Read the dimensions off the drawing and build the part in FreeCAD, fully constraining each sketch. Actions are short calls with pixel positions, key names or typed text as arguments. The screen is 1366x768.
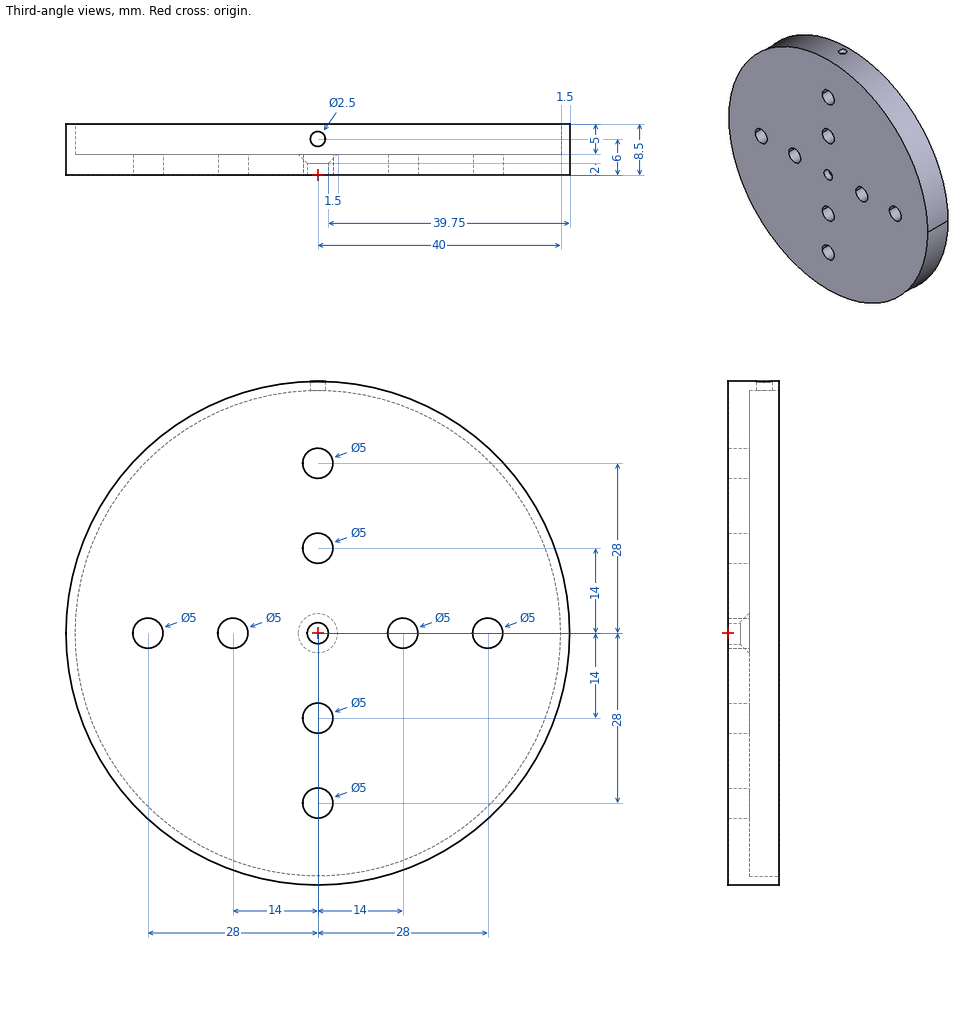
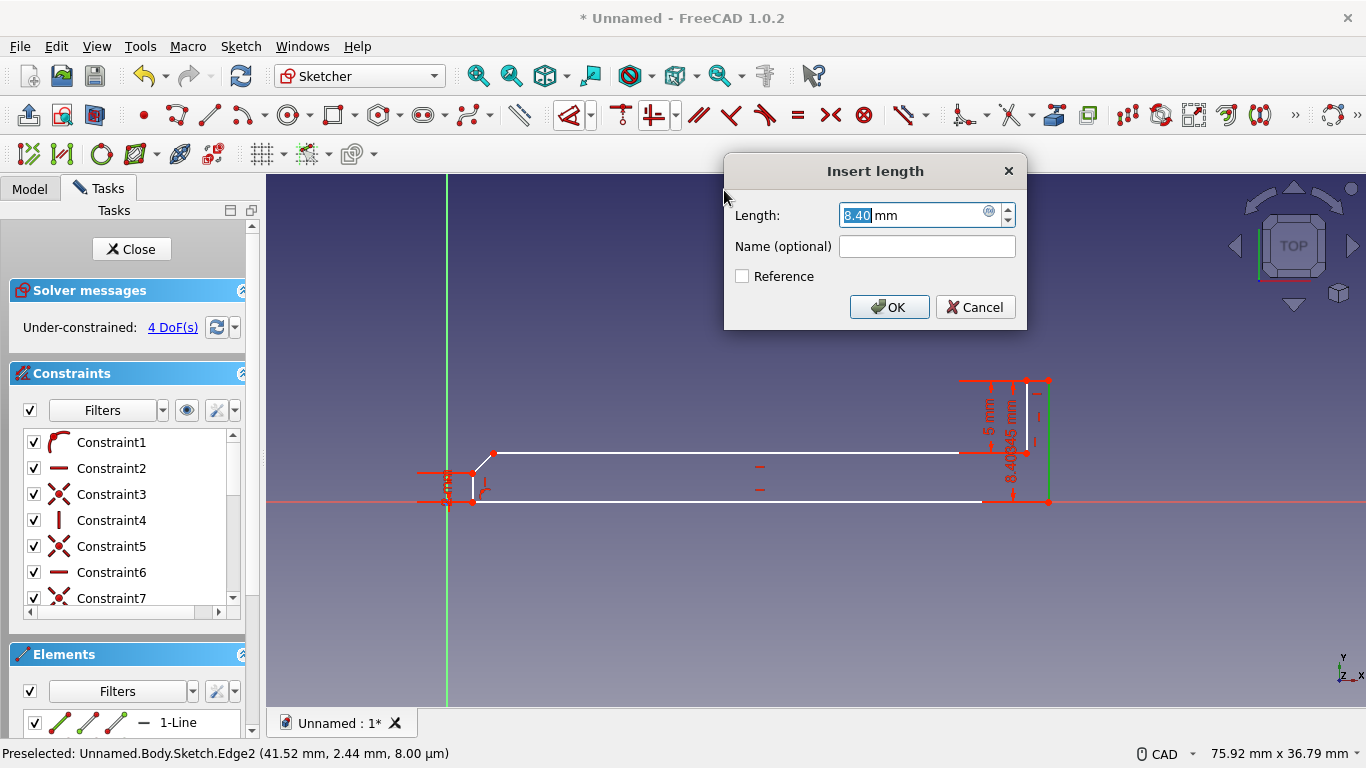
text(8.5)
key(Return)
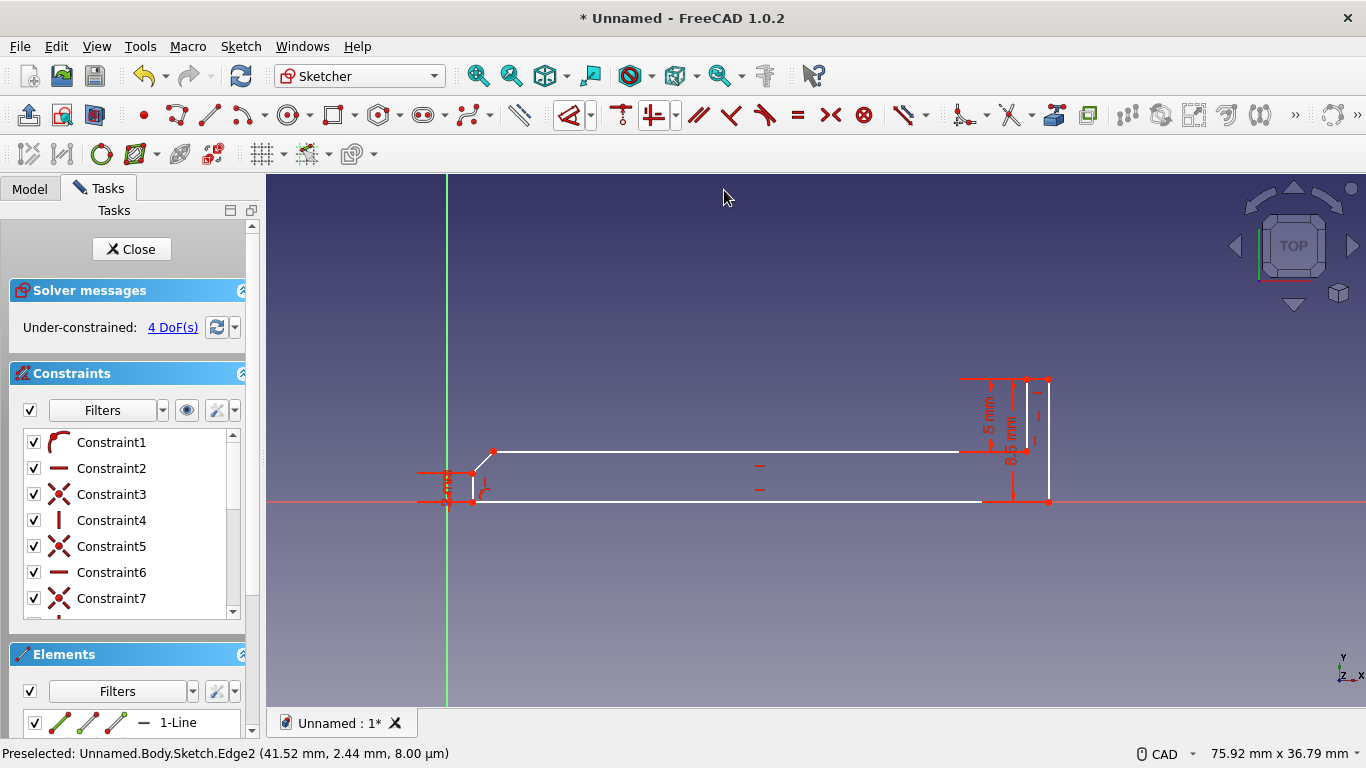
scroll(1038, 379, up, 4)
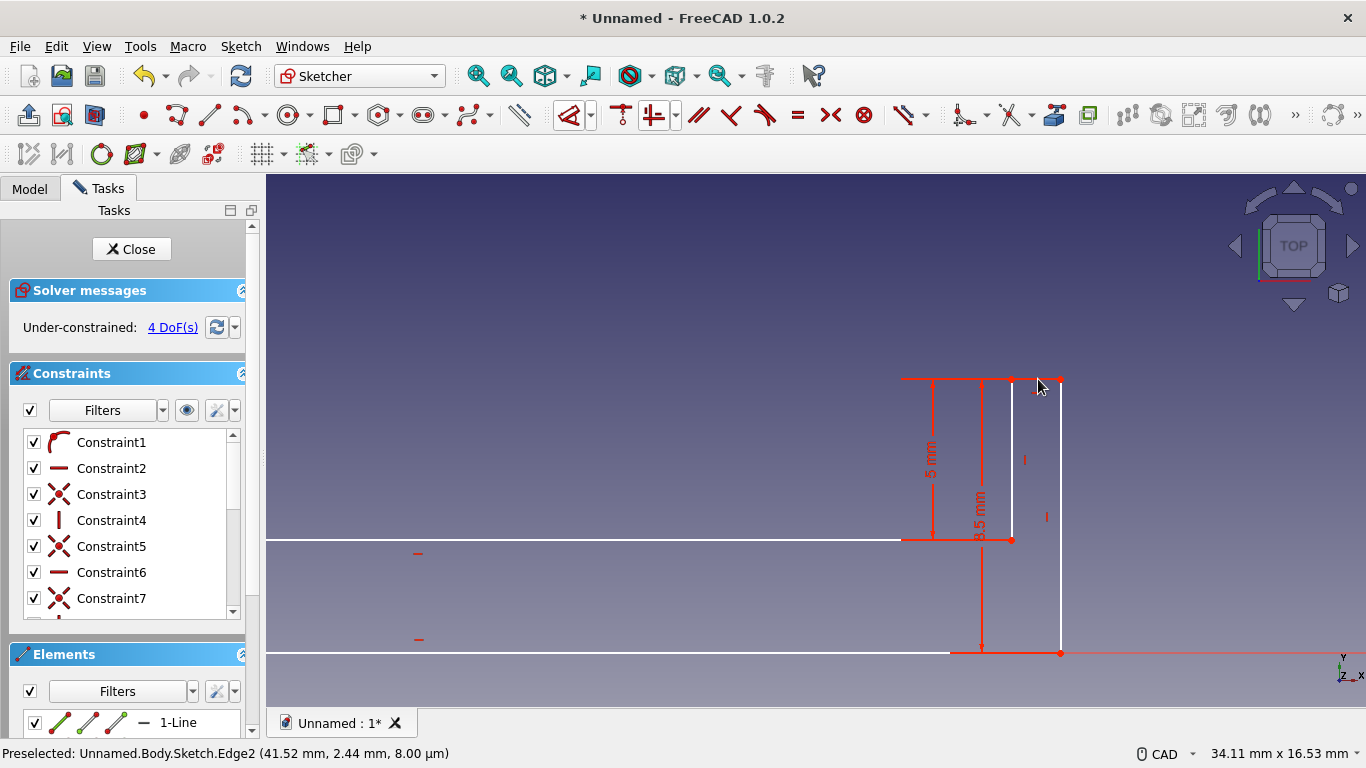
click(1036, 379)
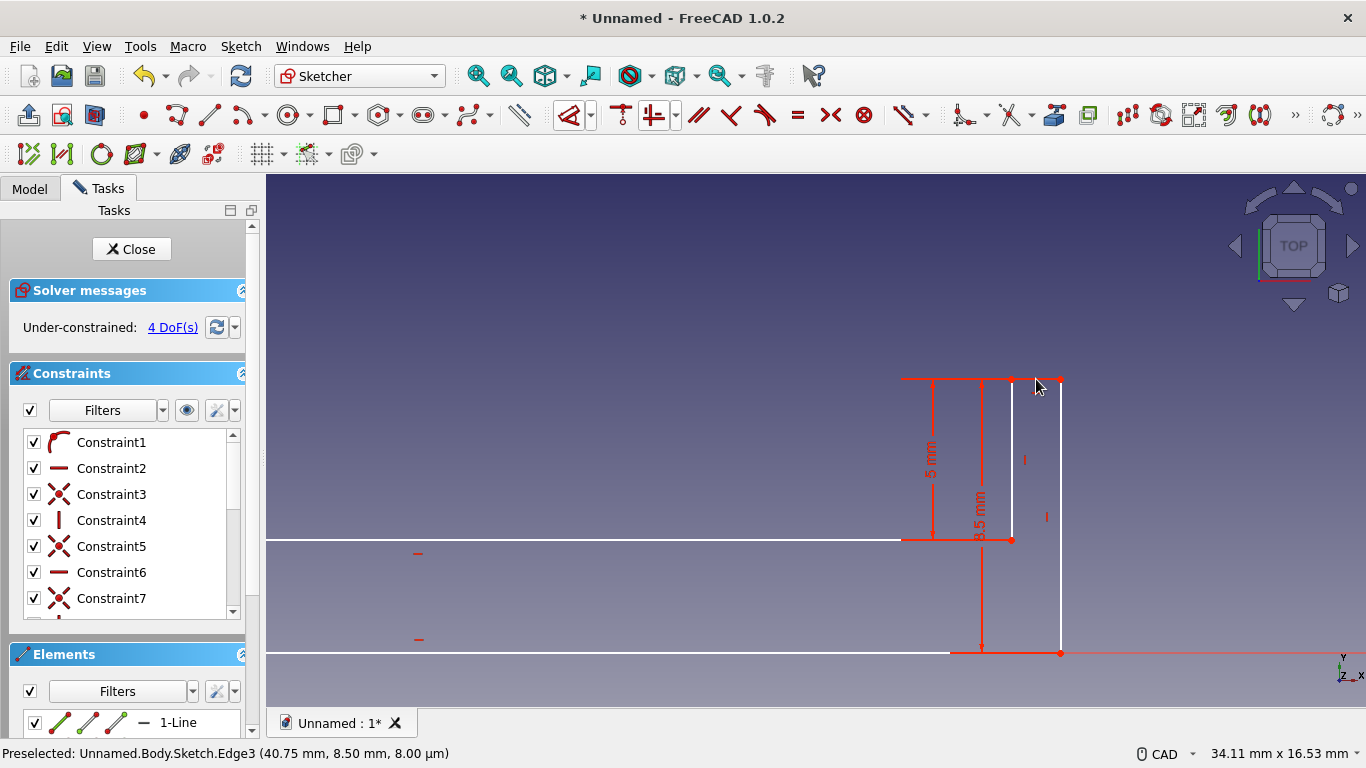
key(l)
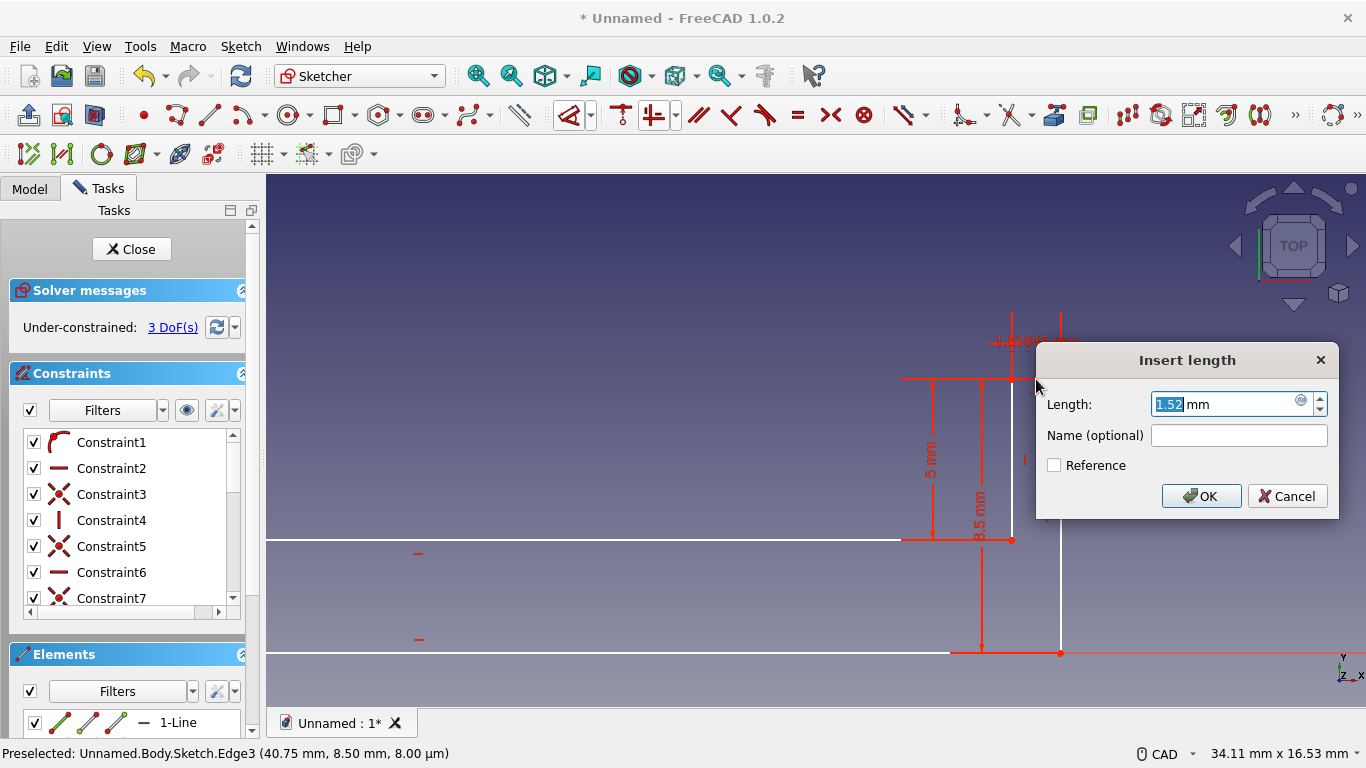
text(1.5)
key(Return)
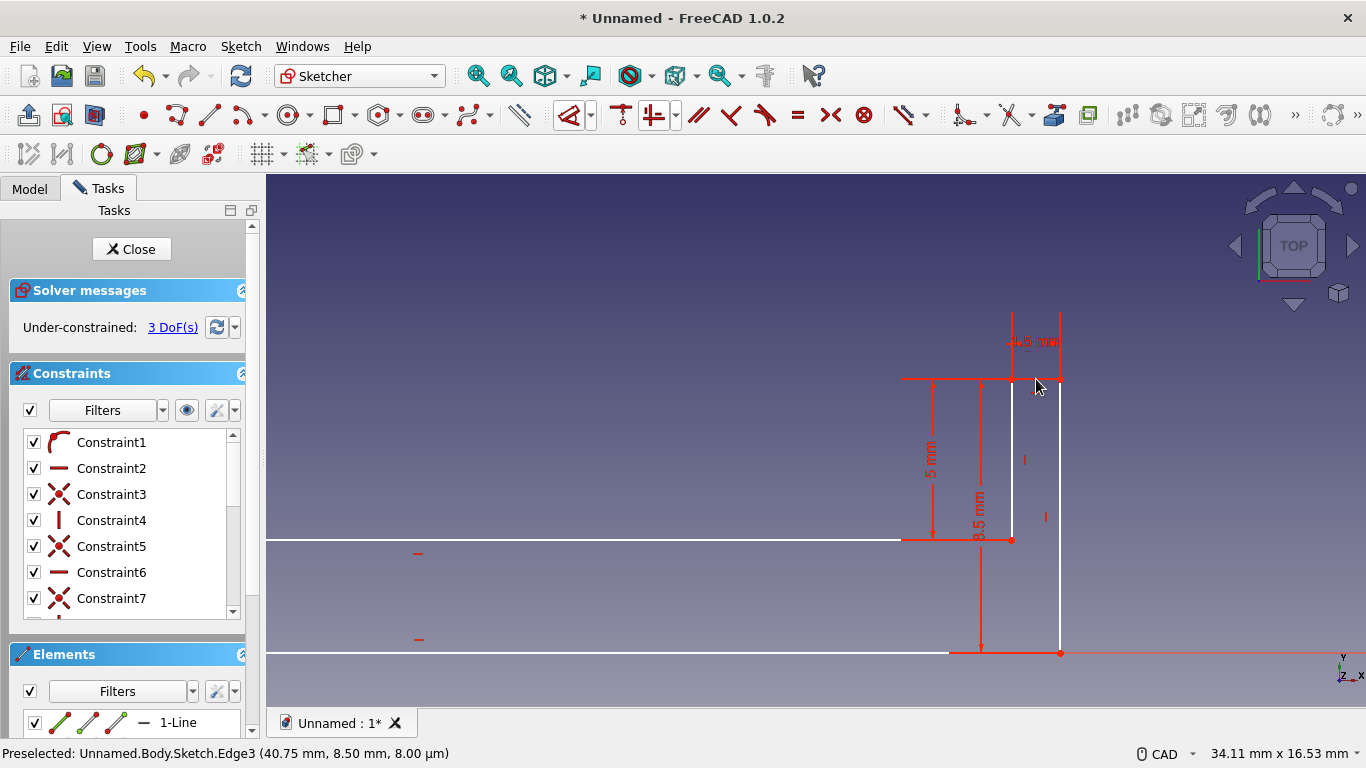
click(1012, 379)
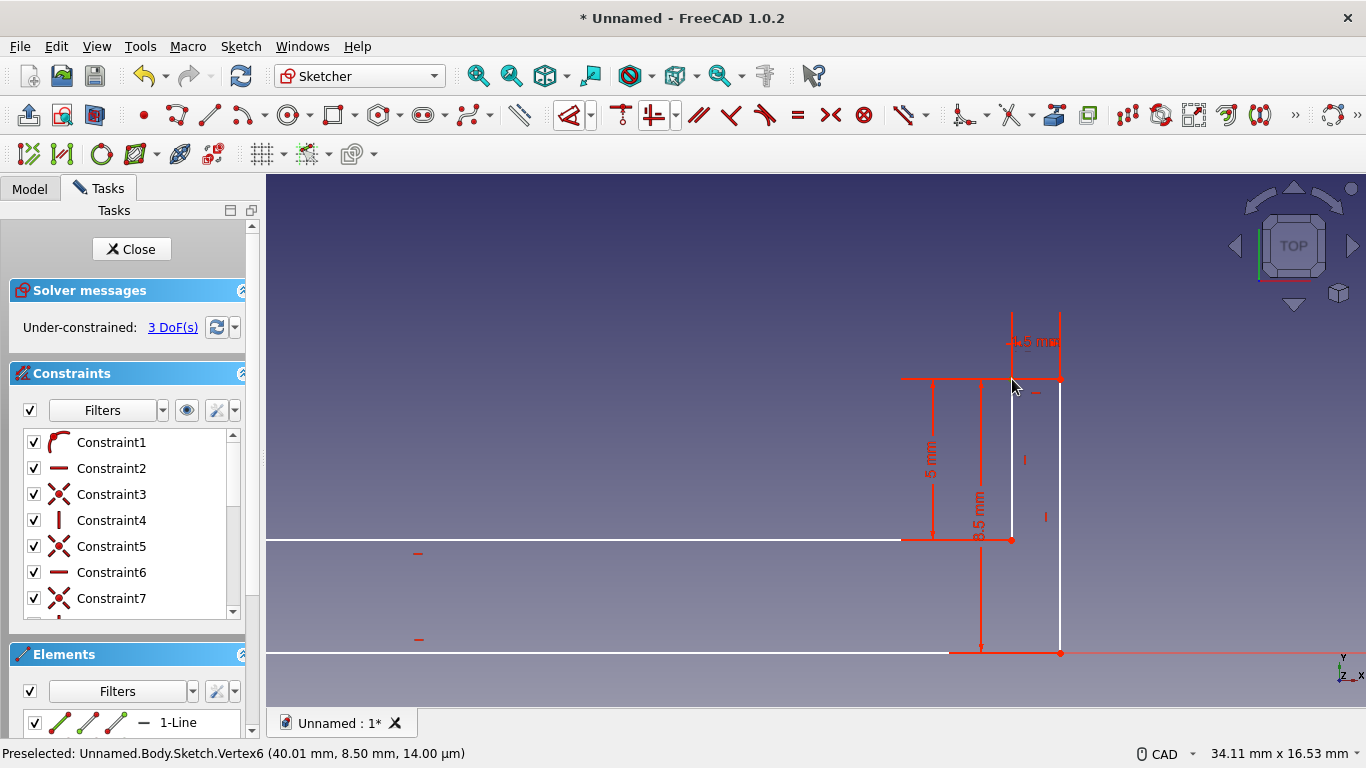
click(590, 116)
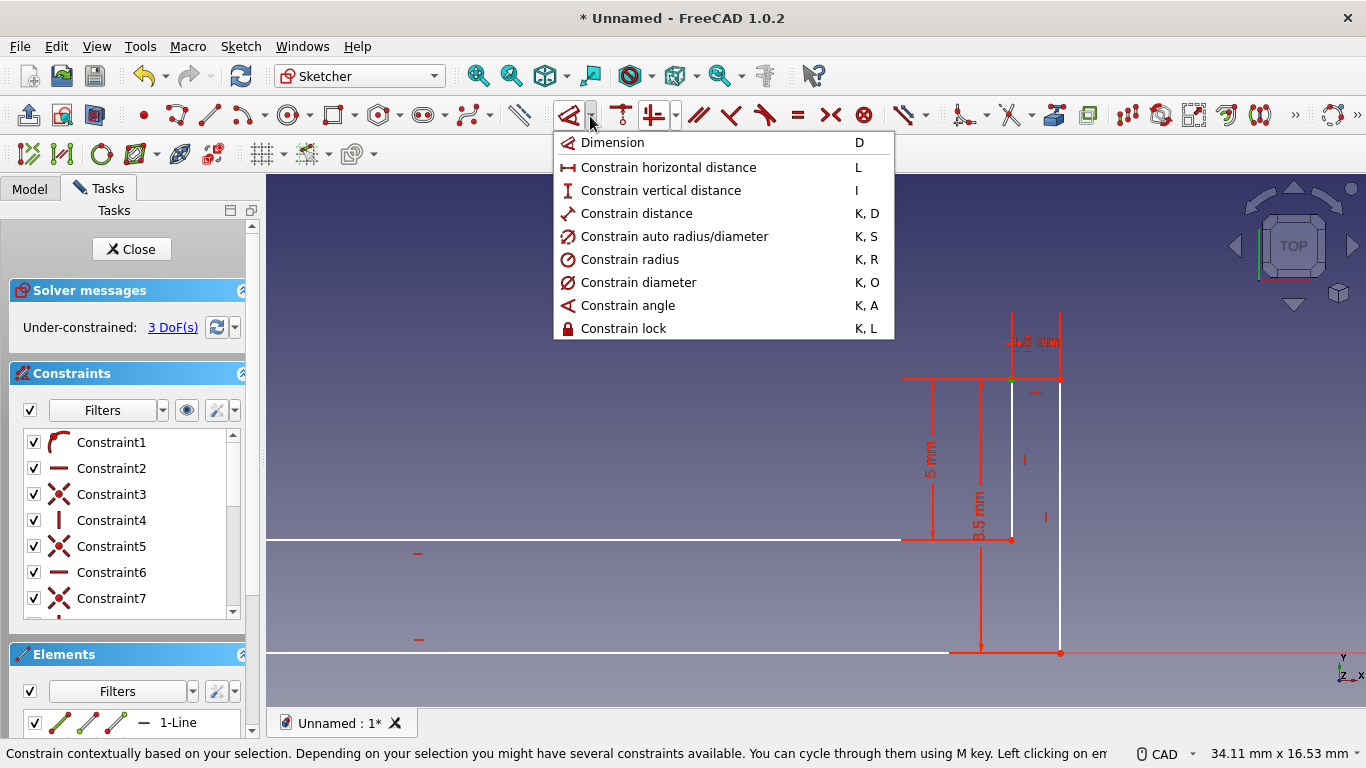
click(724, 168)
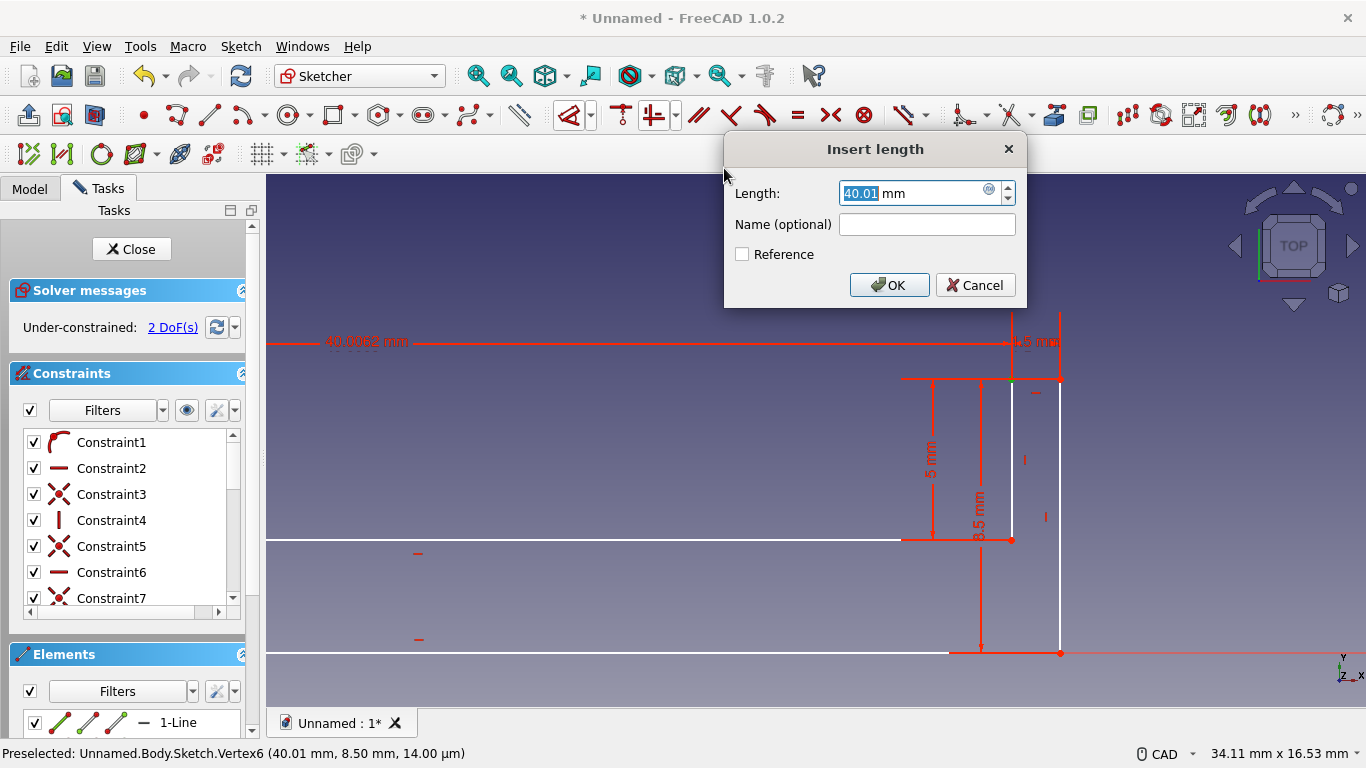
text(40)
key(Return)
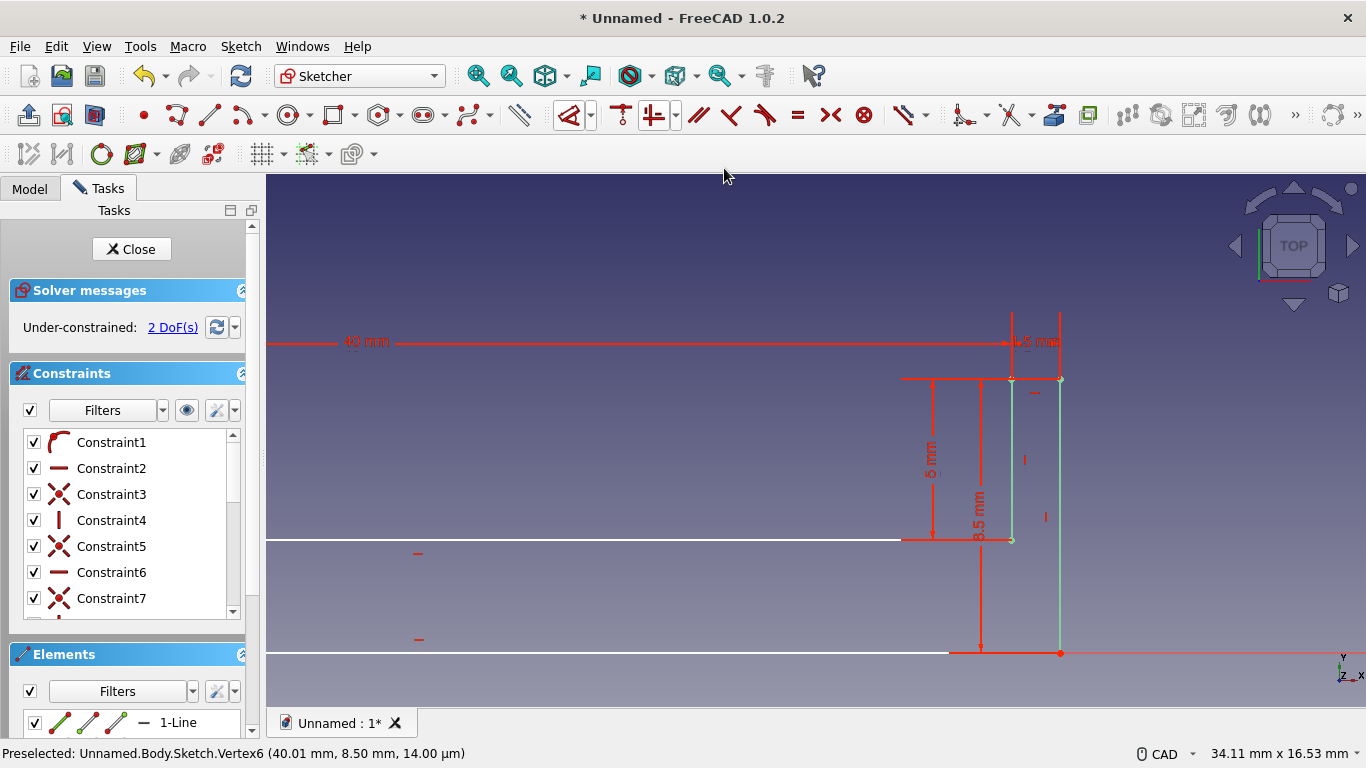
scroll(1038, 379, down, 4)